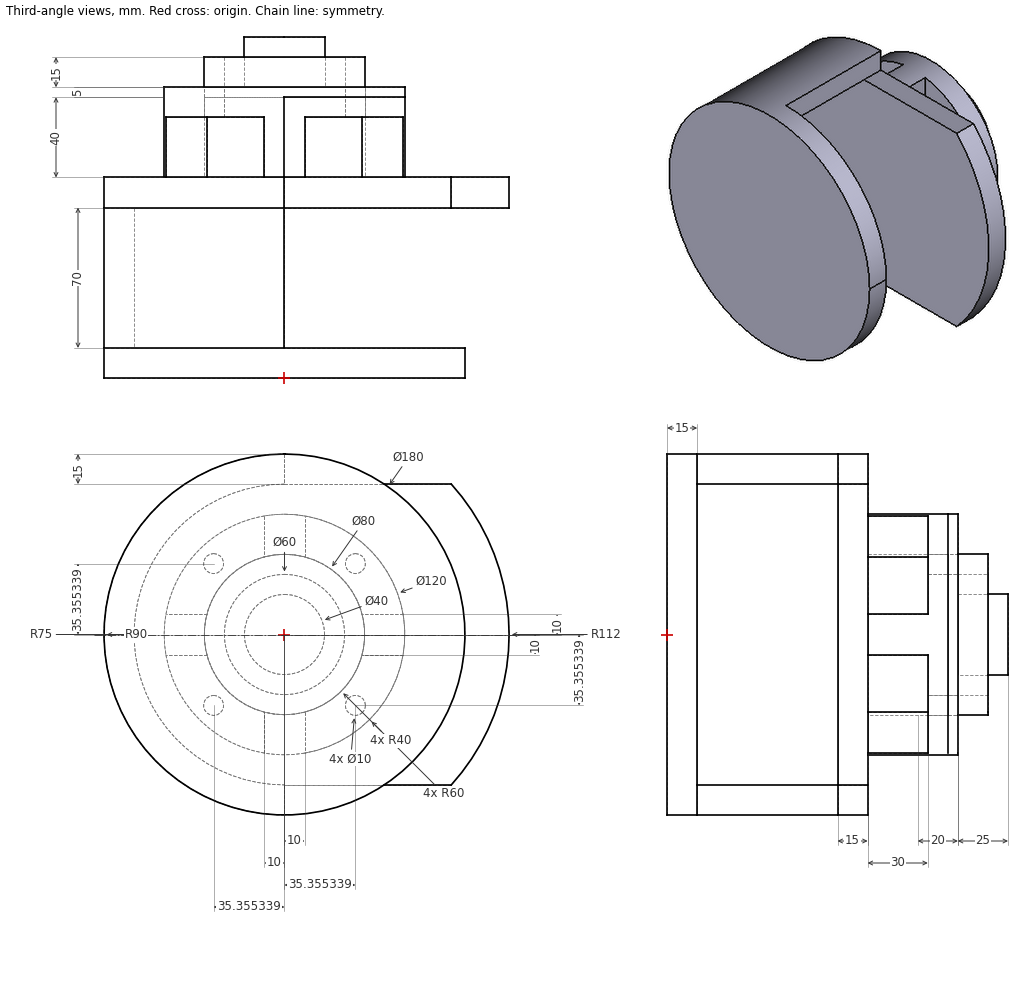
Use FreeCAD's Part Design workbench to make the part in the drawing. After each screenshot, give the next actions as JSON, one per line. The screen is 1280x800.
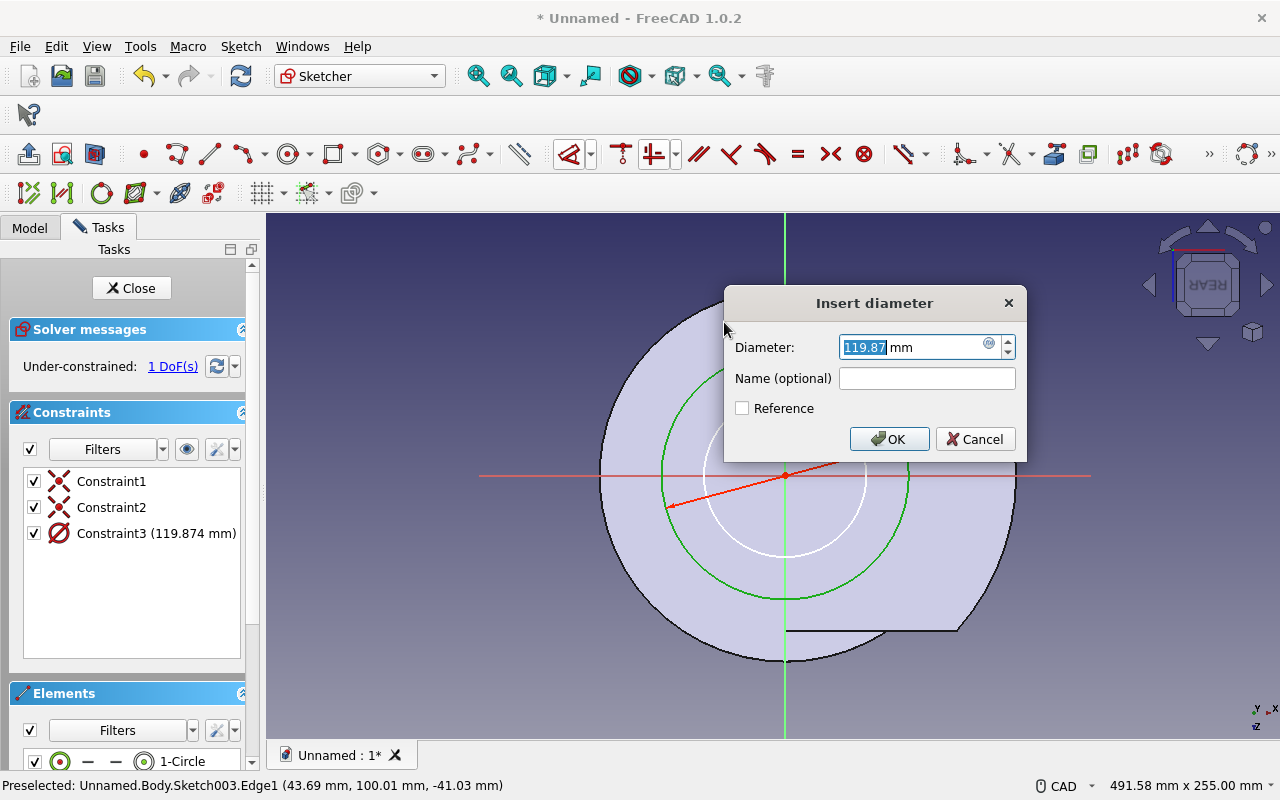
{"action": "type", "text": "120"}
{"action": "key", "text": "Return"}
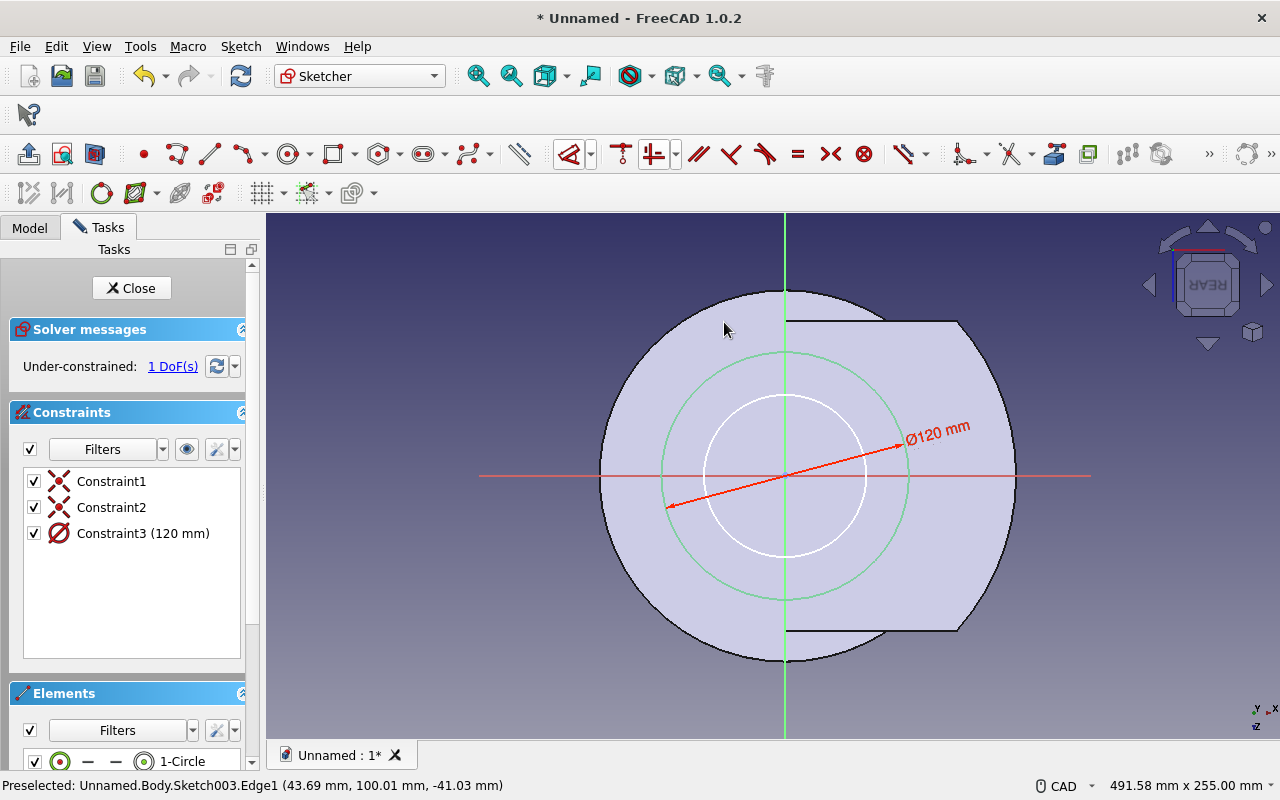
{"action": "left_click", "coordinate": [842, 418]}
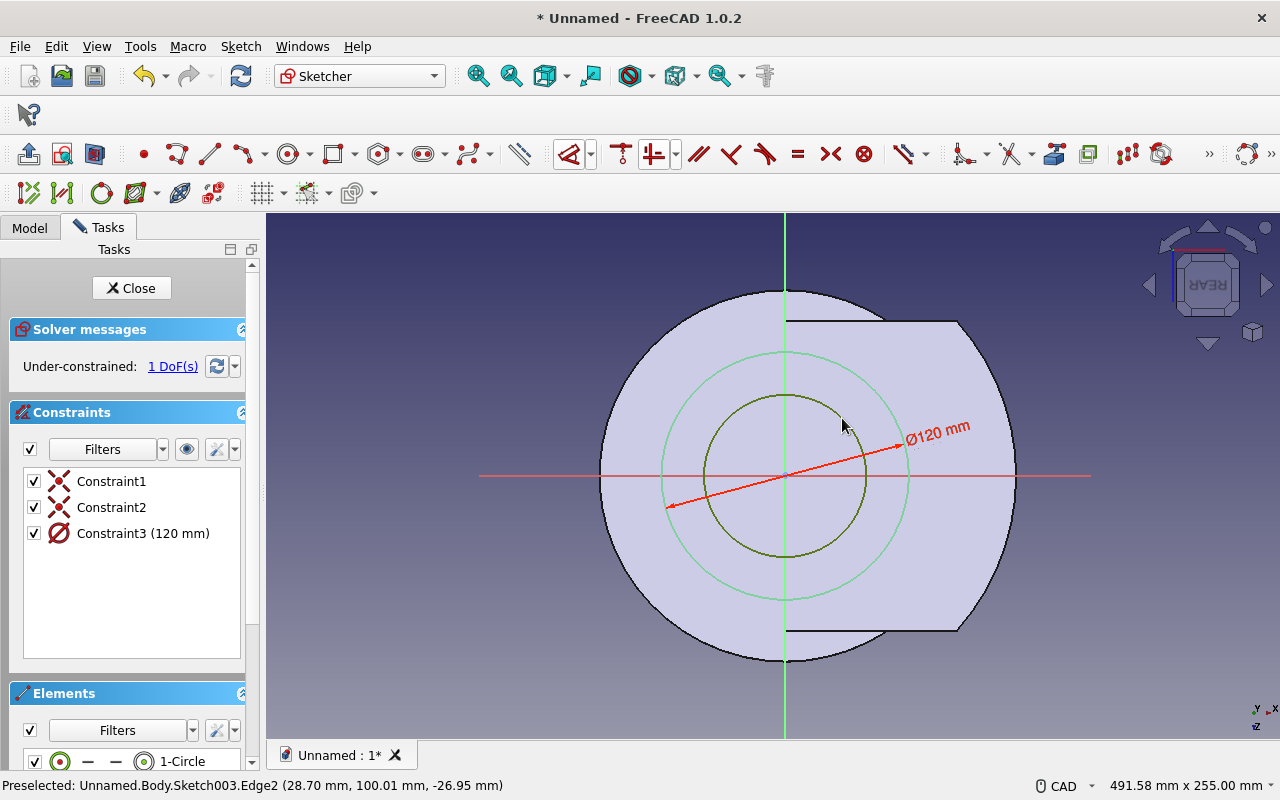
{"action": "left_click", "coordinate": [590, 154]}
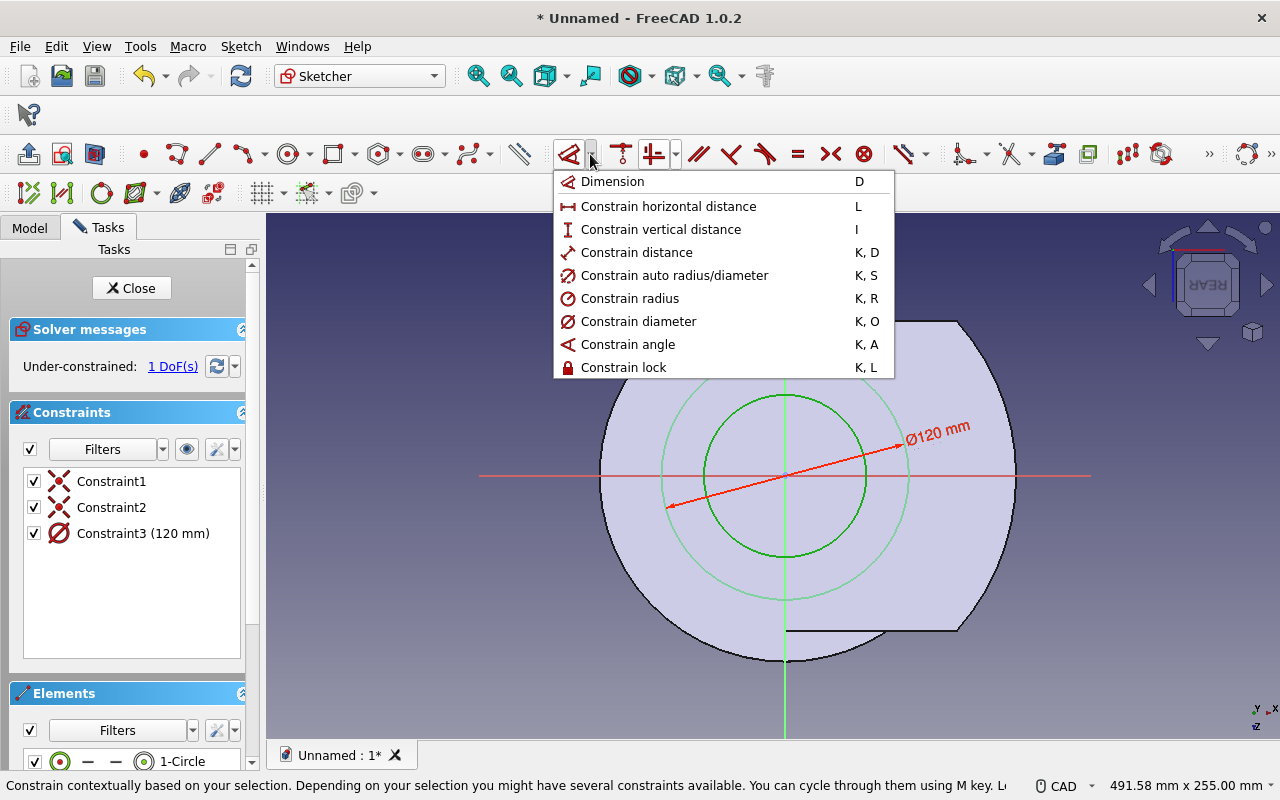
{"action": "left_click", "coordinate": [724, 322]}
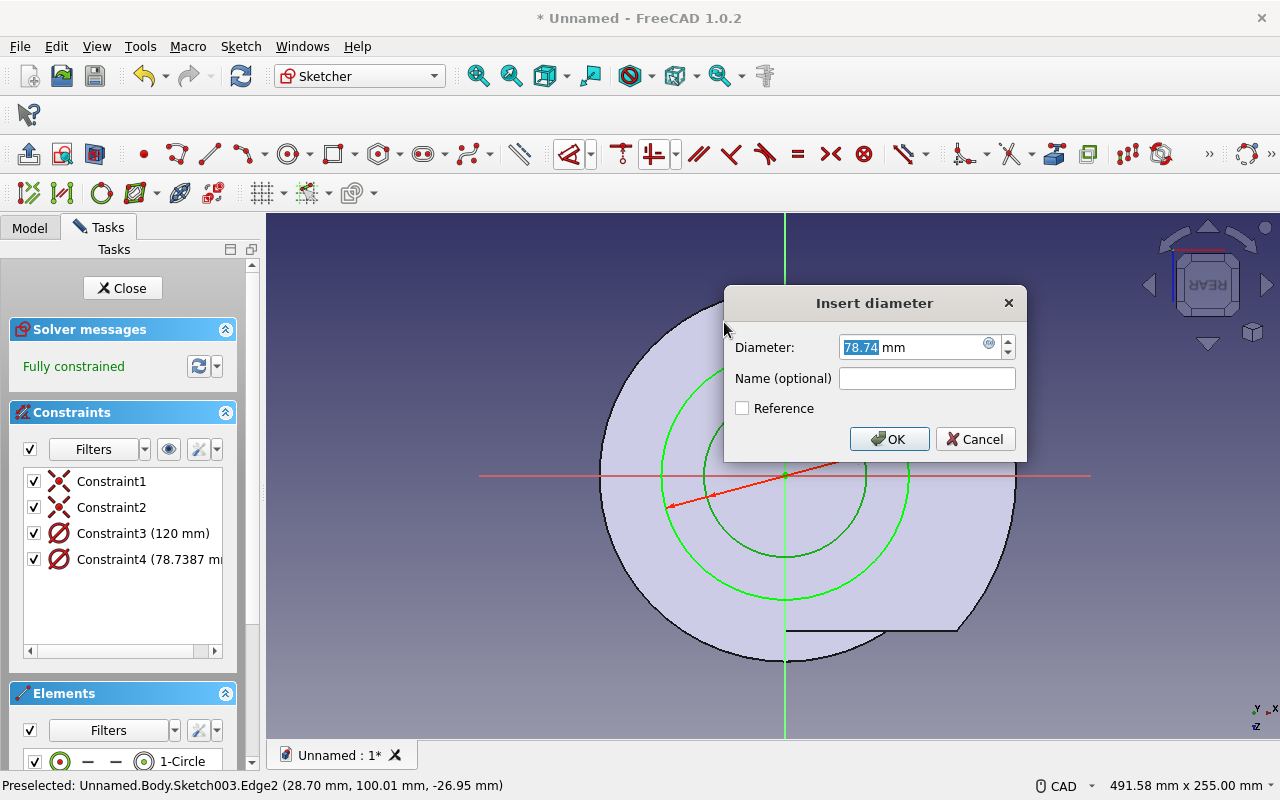
{"action": "type", "text": "80"}
{"action": "key", "text": "Return"}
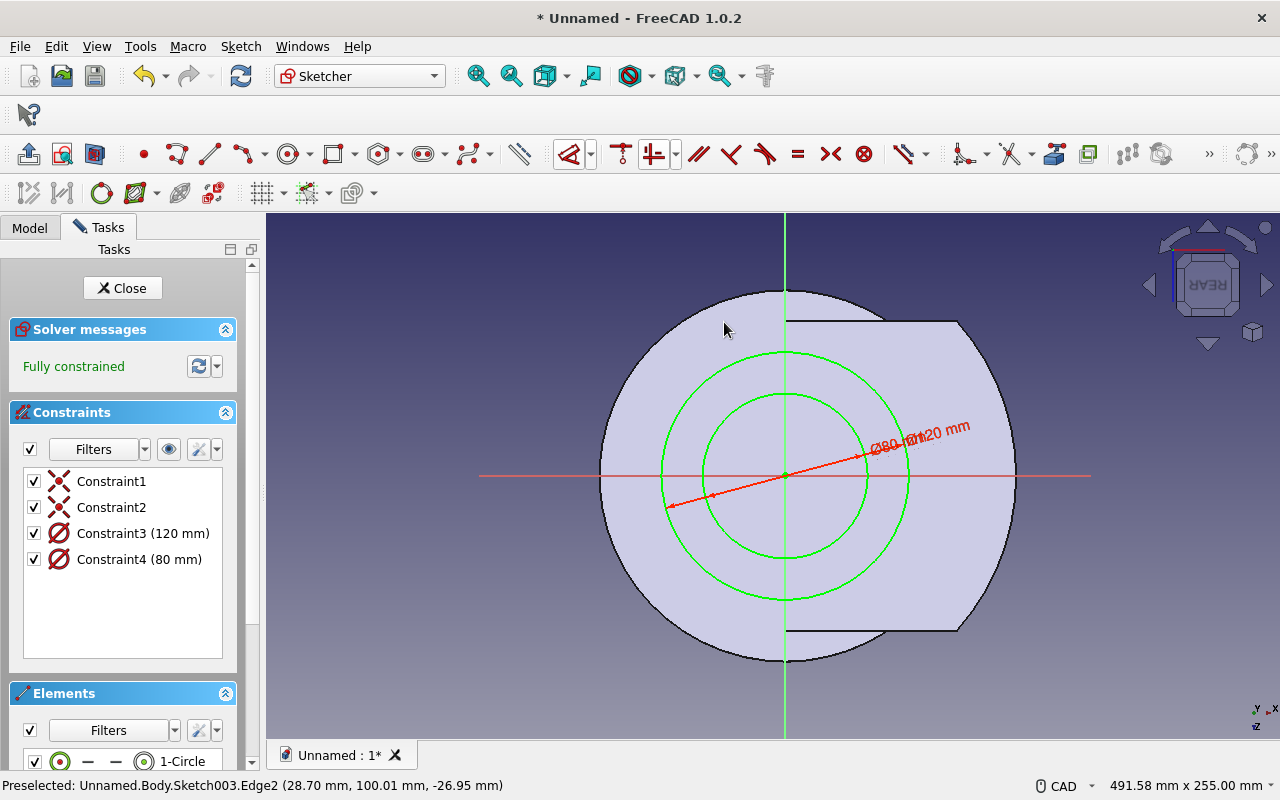
{"action": "left_click", "coordinate": [123, 288]}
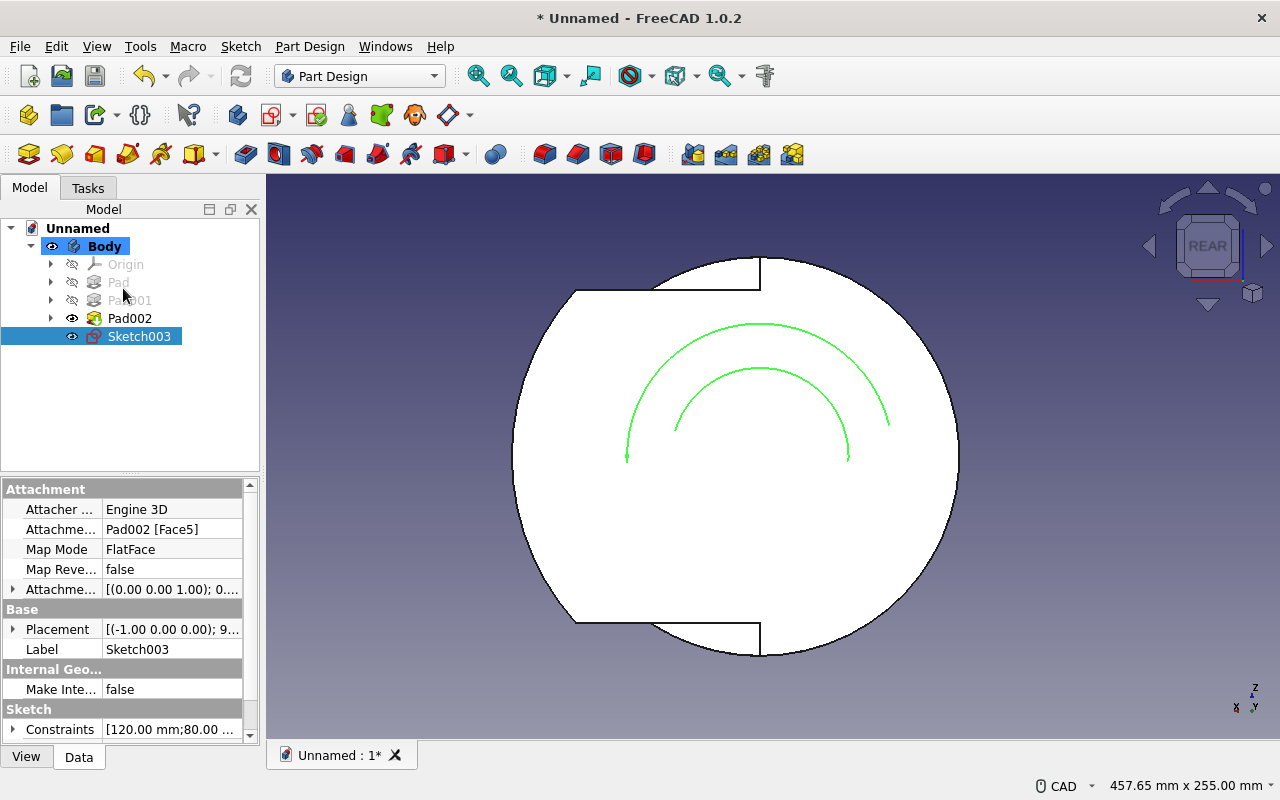
{"action": "left_click", "coordinate": [29, 154]}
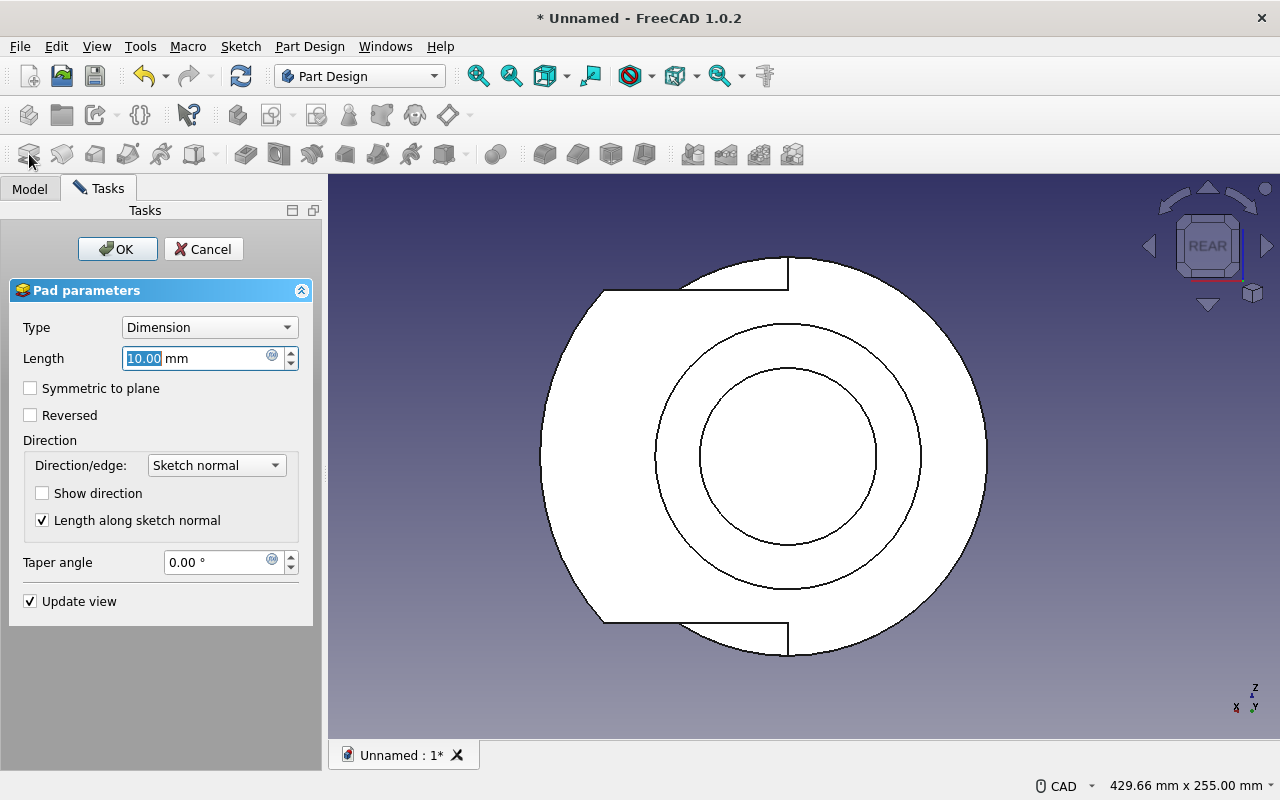
{"action": "type", "text": "40"}
{"action": "key", "text": "Tab"}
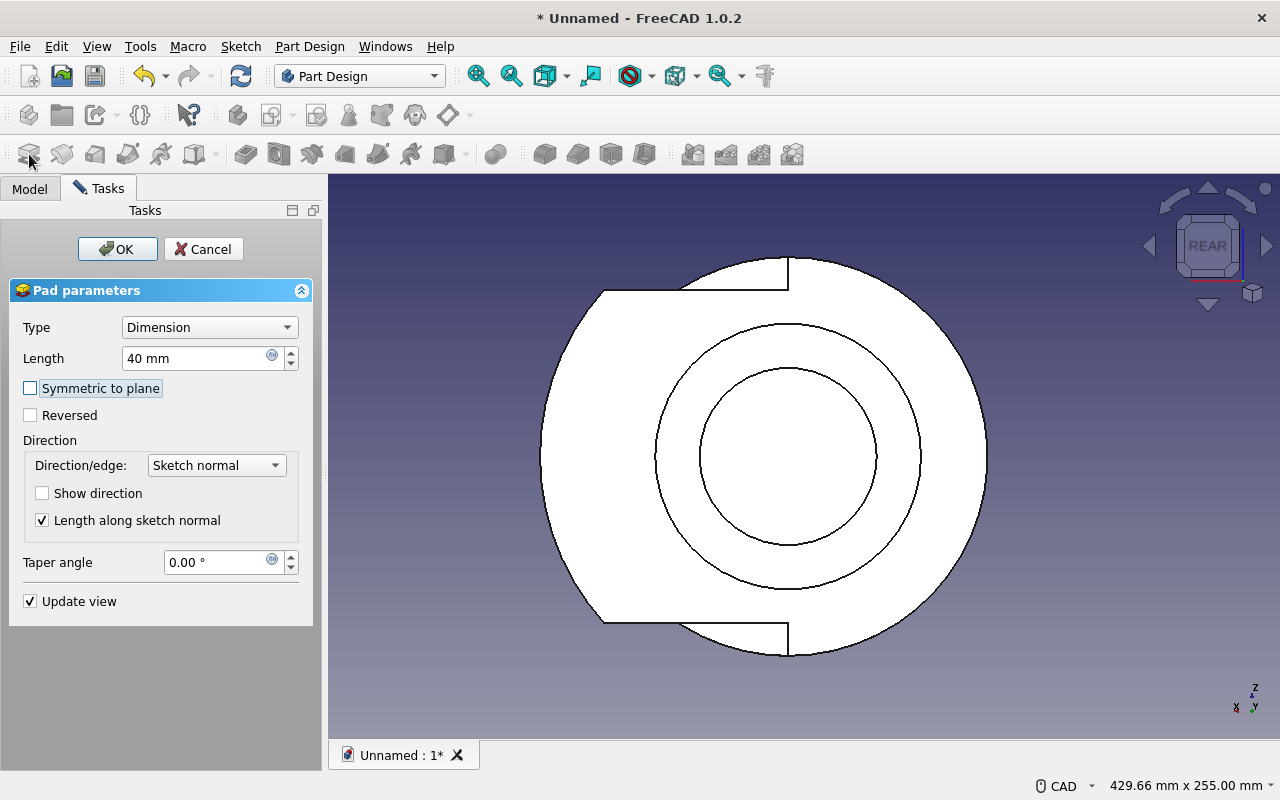
{"action": "left_click", "coordinate": [118, 249]}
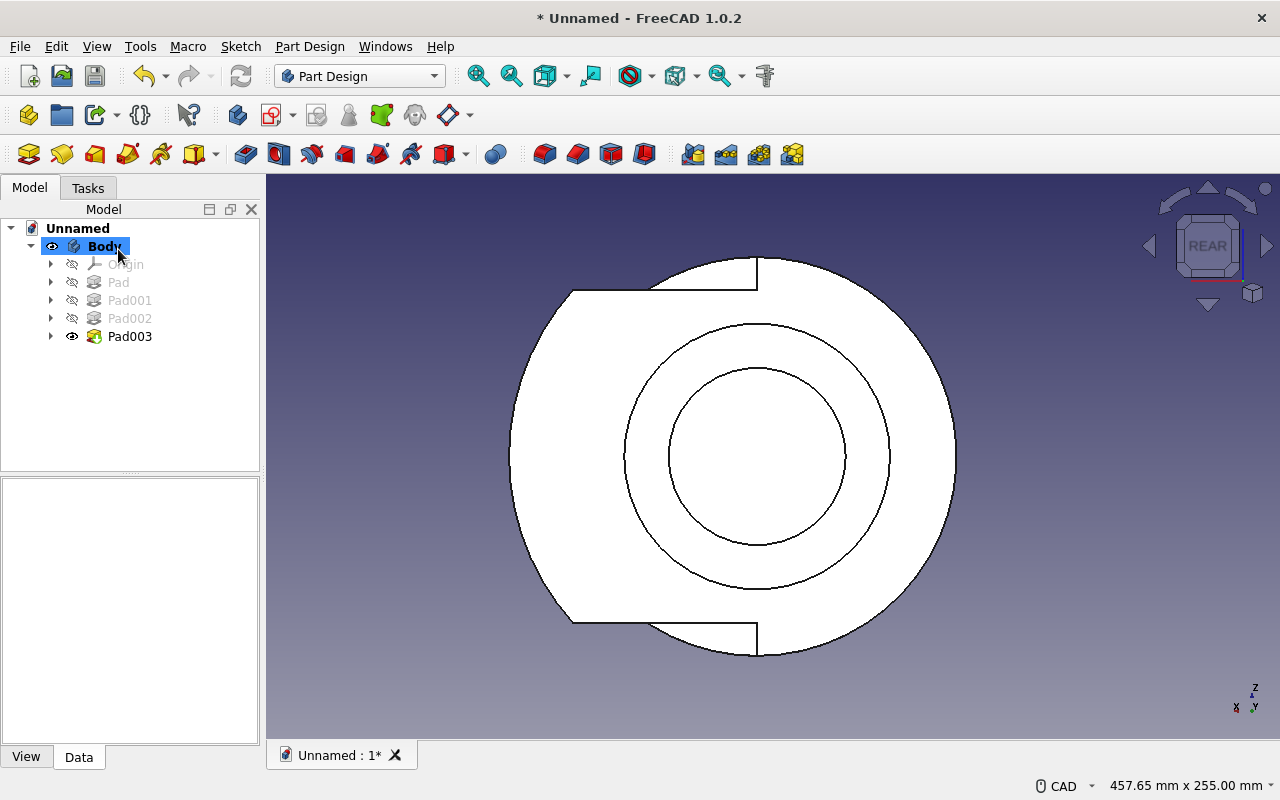
{"action": "left_click", "coordinate": [605, 342]}